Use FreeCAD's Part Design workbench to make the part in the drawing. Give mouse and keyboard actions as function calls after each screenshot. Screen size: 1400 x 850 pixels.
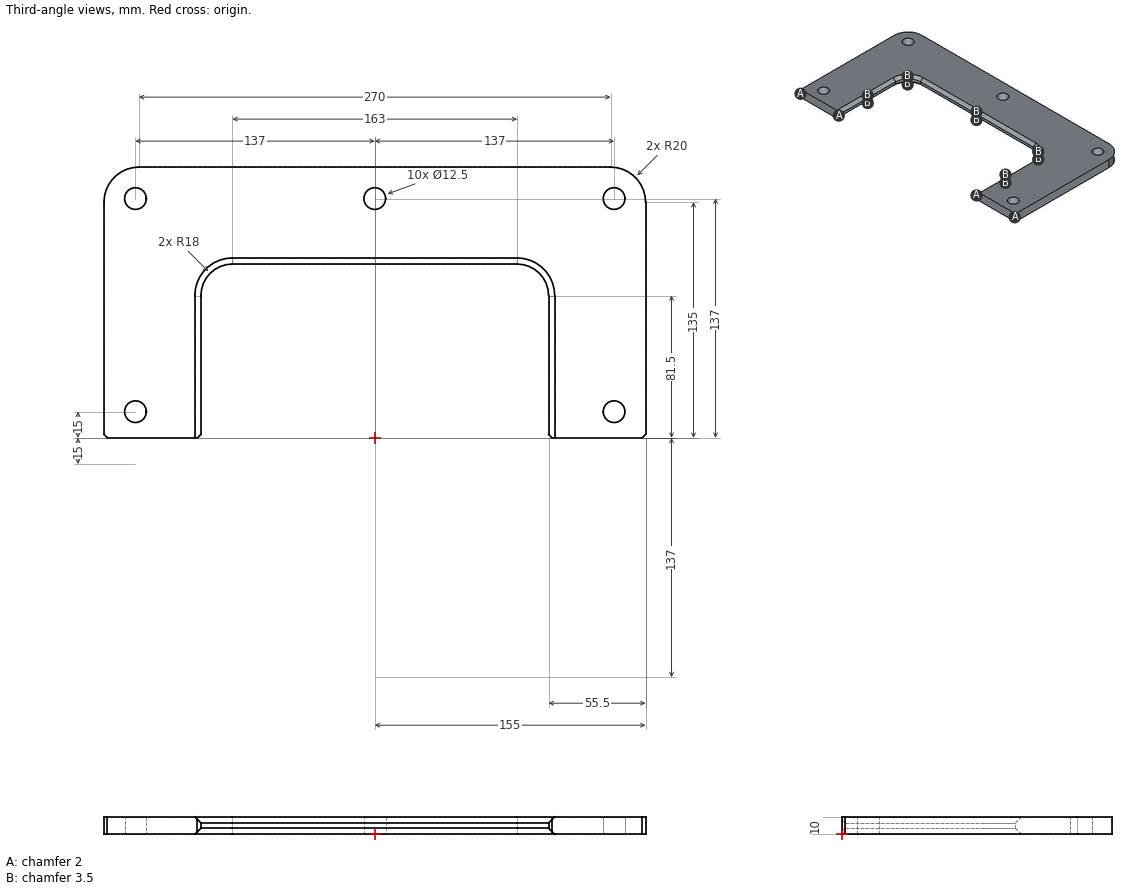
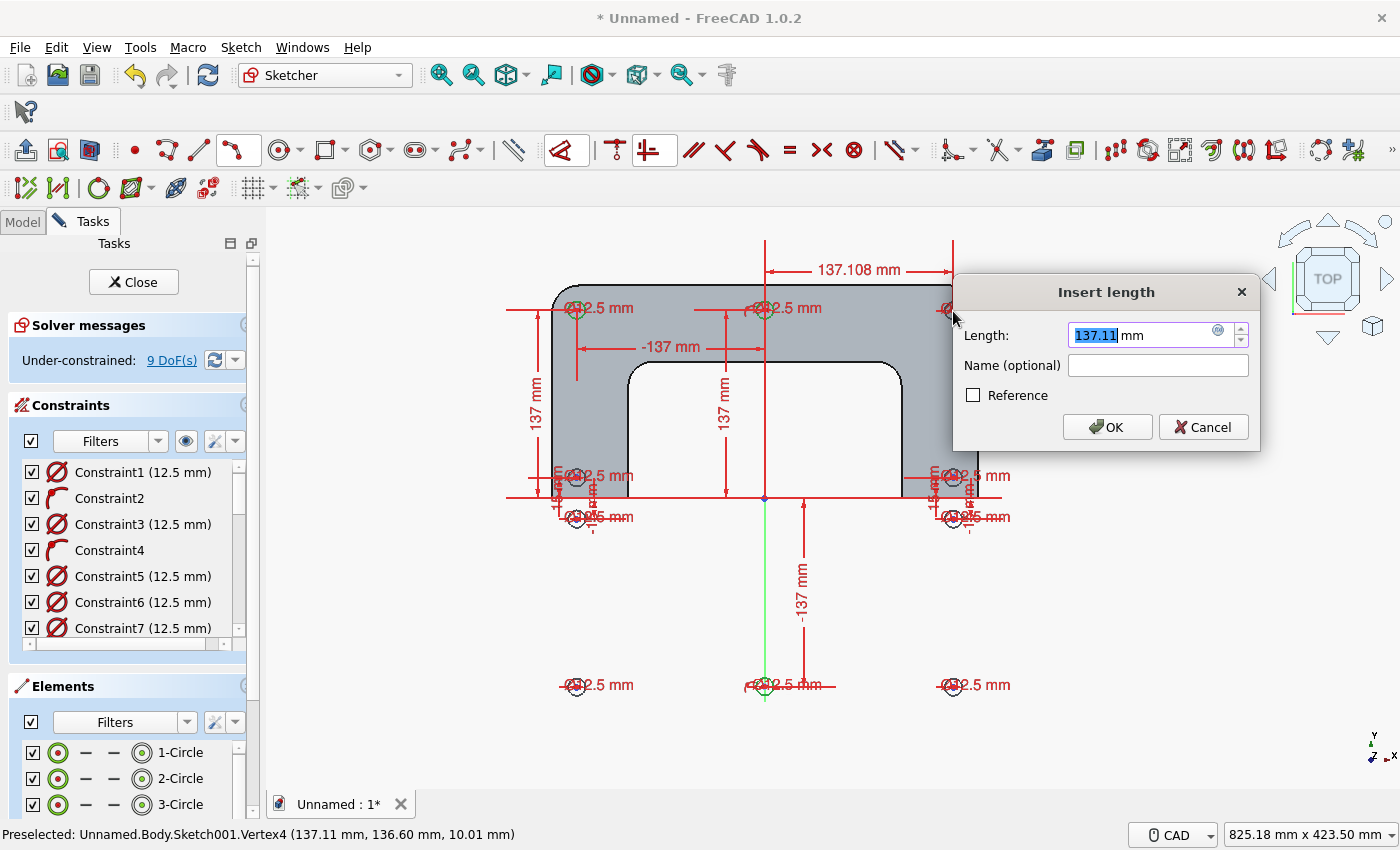
text(137)
key(Return)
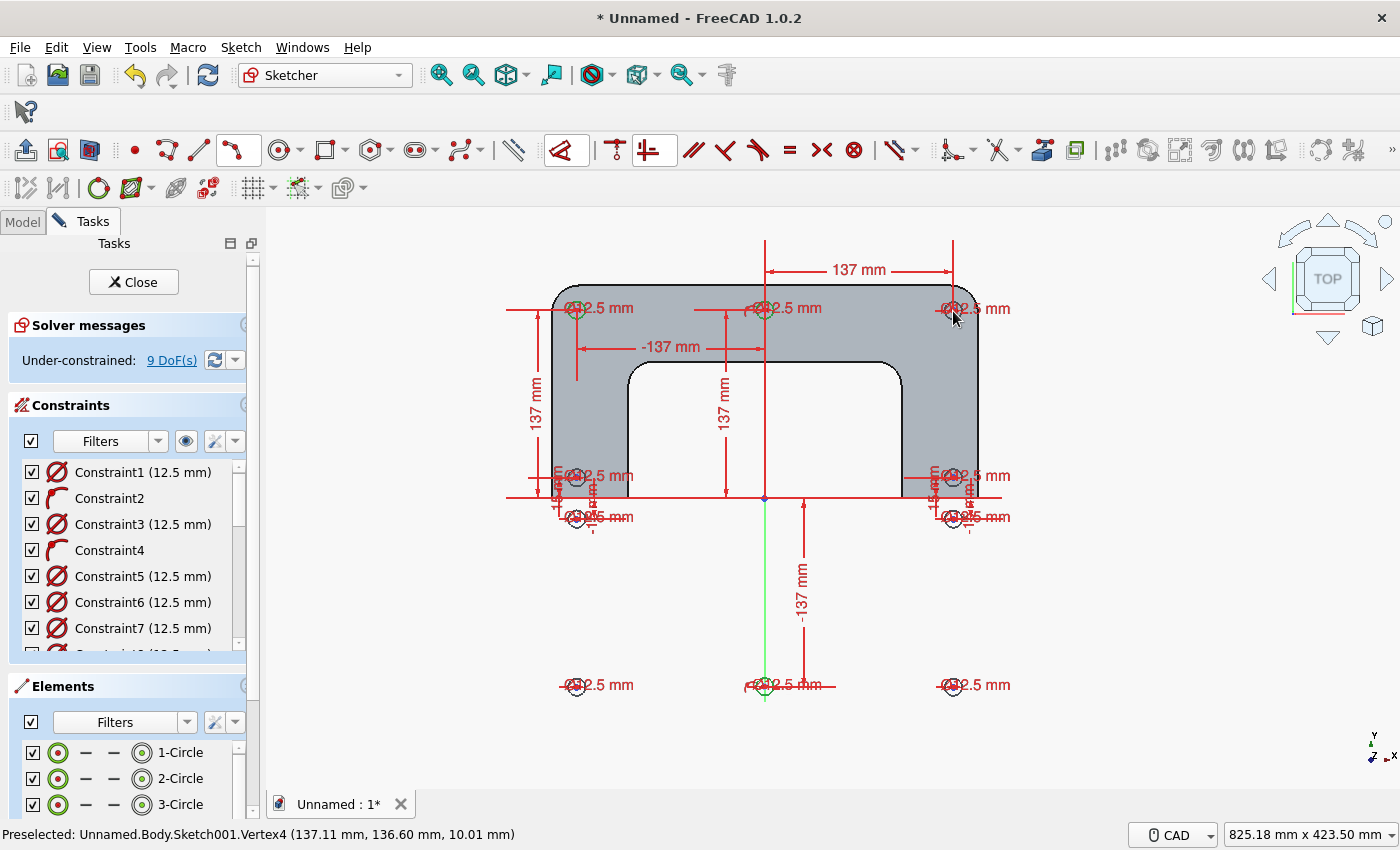
click(953, 311)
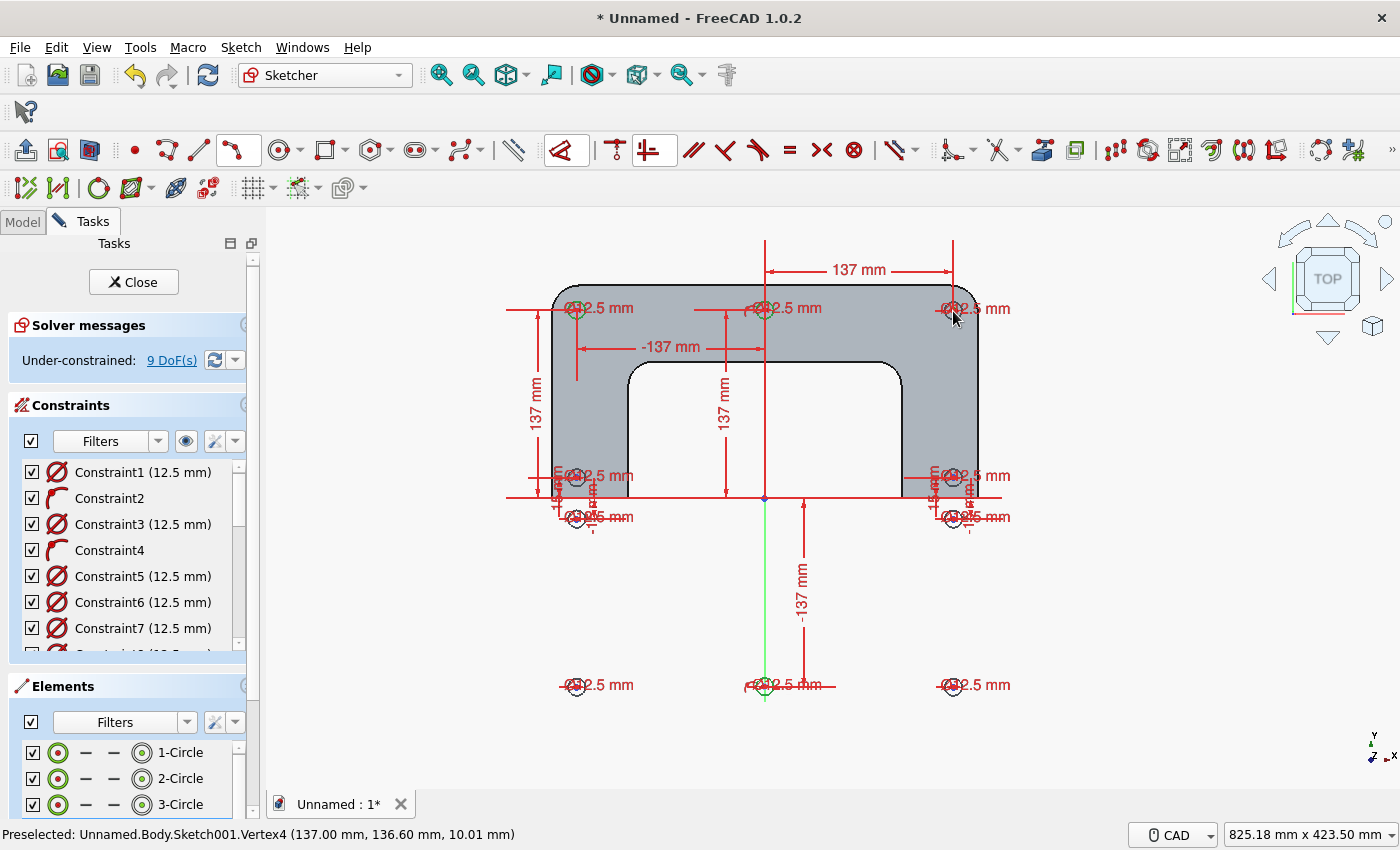
key(i)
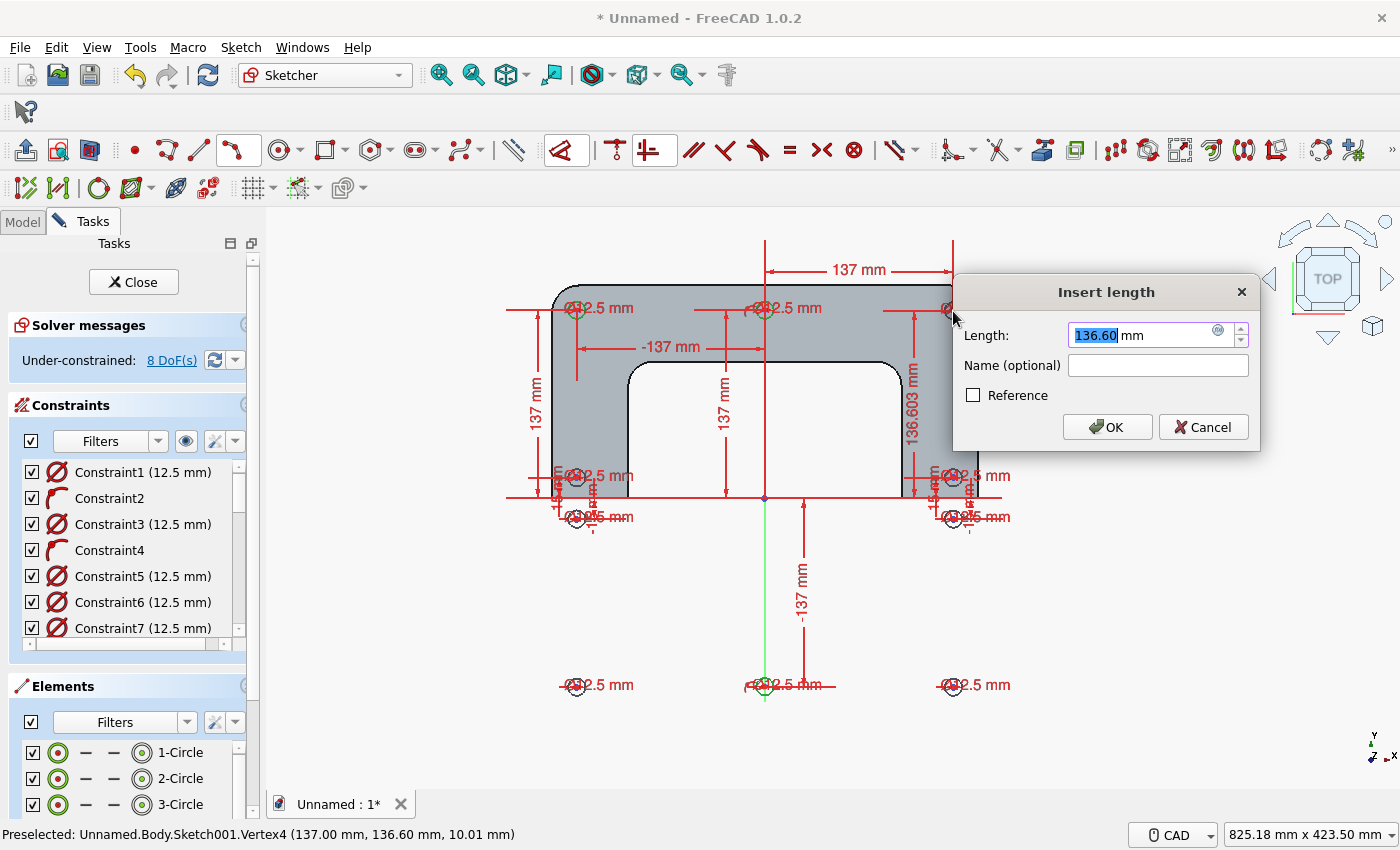
text(137)
key(Return)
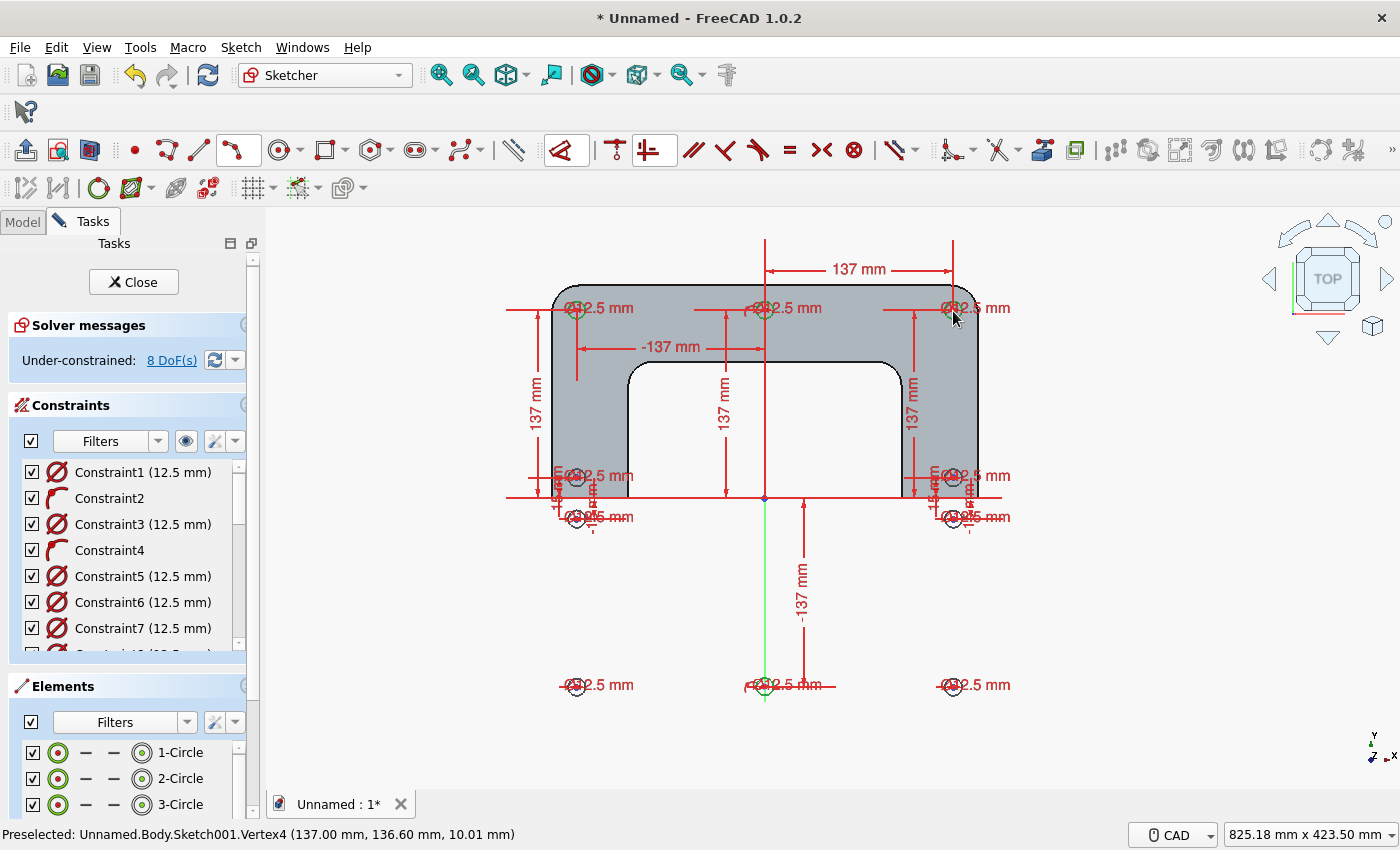
click(577, 687)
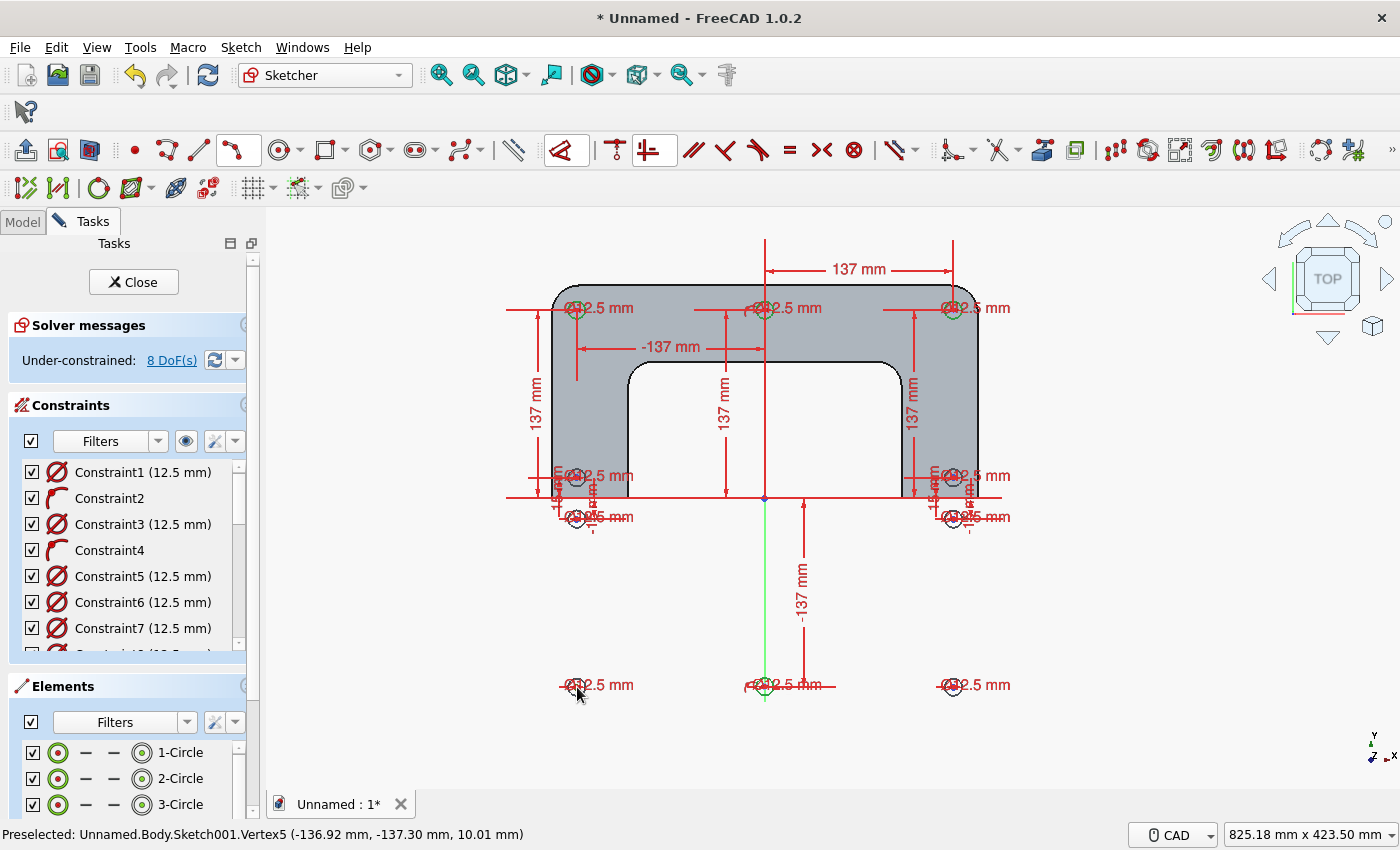
key(l)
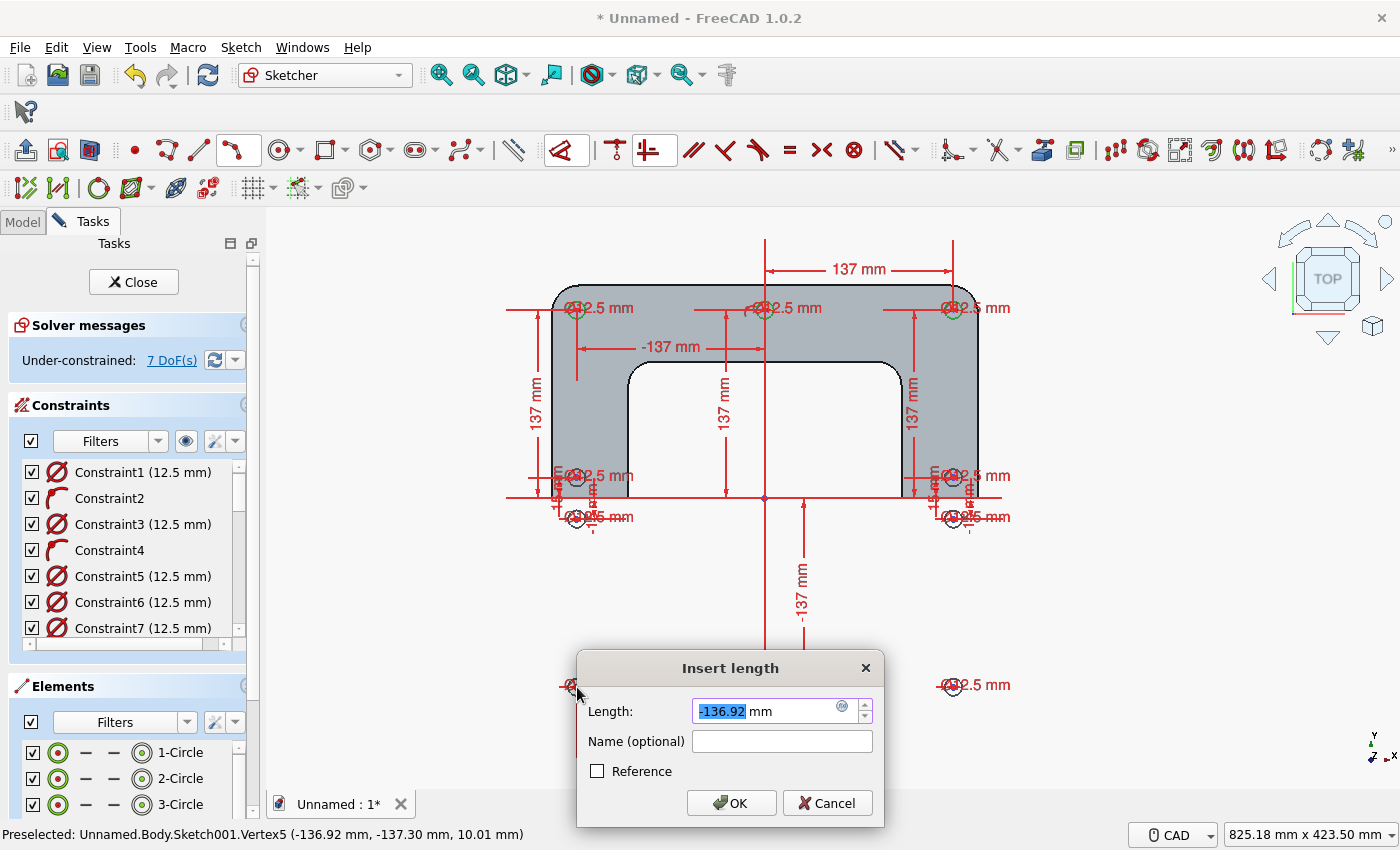
text(-137)
key(Return)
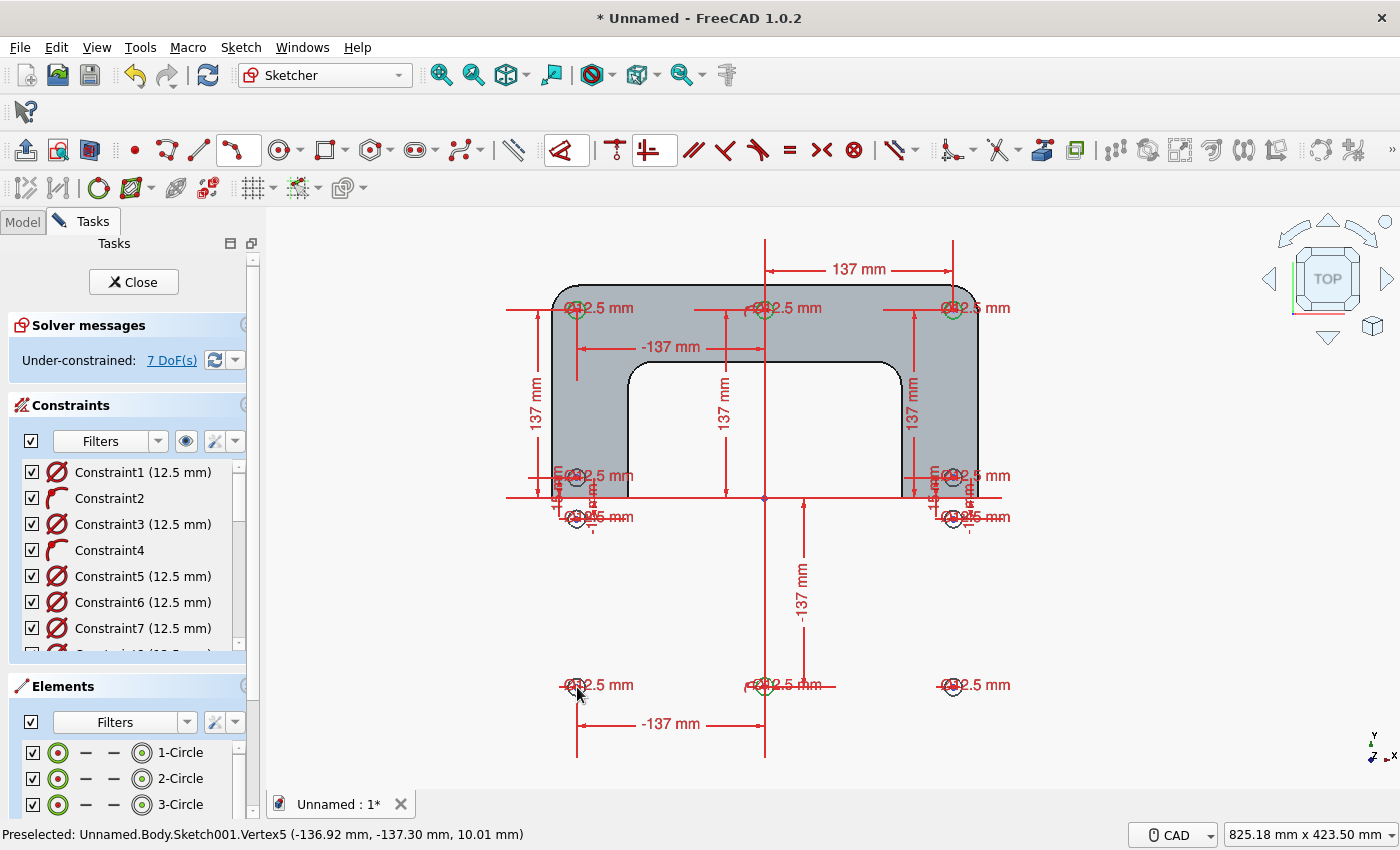
click(577, 687)